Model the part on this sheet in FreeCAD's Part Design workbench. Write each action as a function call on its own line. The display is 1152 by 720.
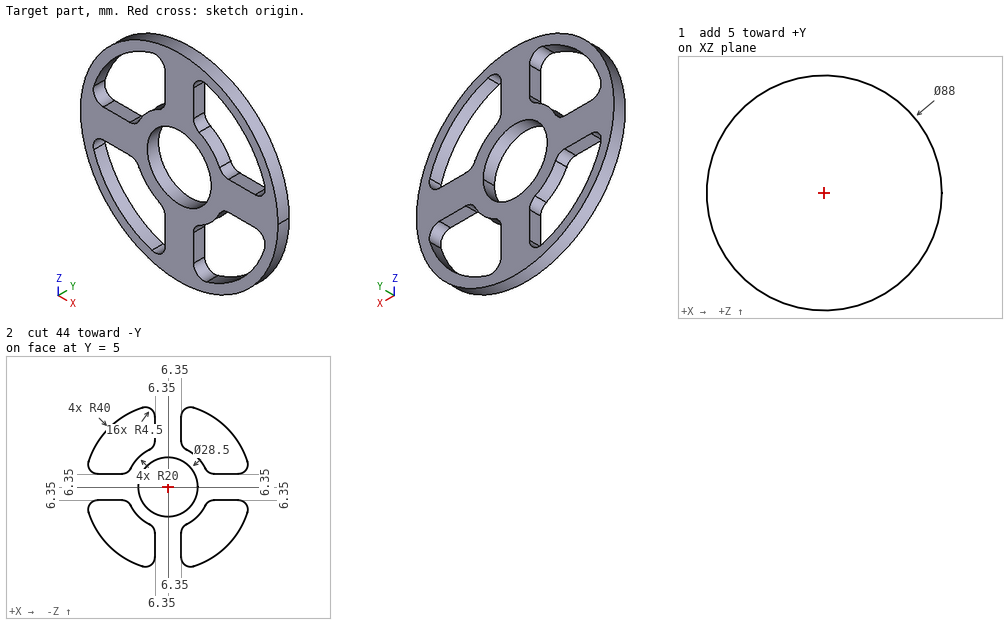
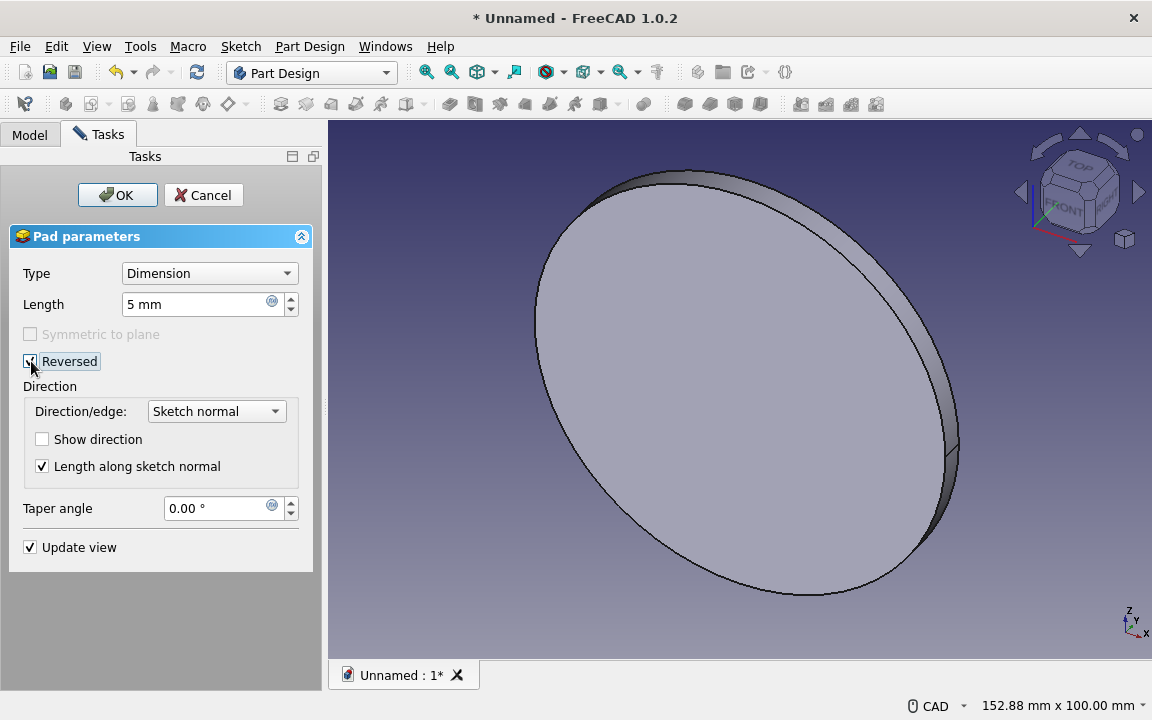
click(118, 195)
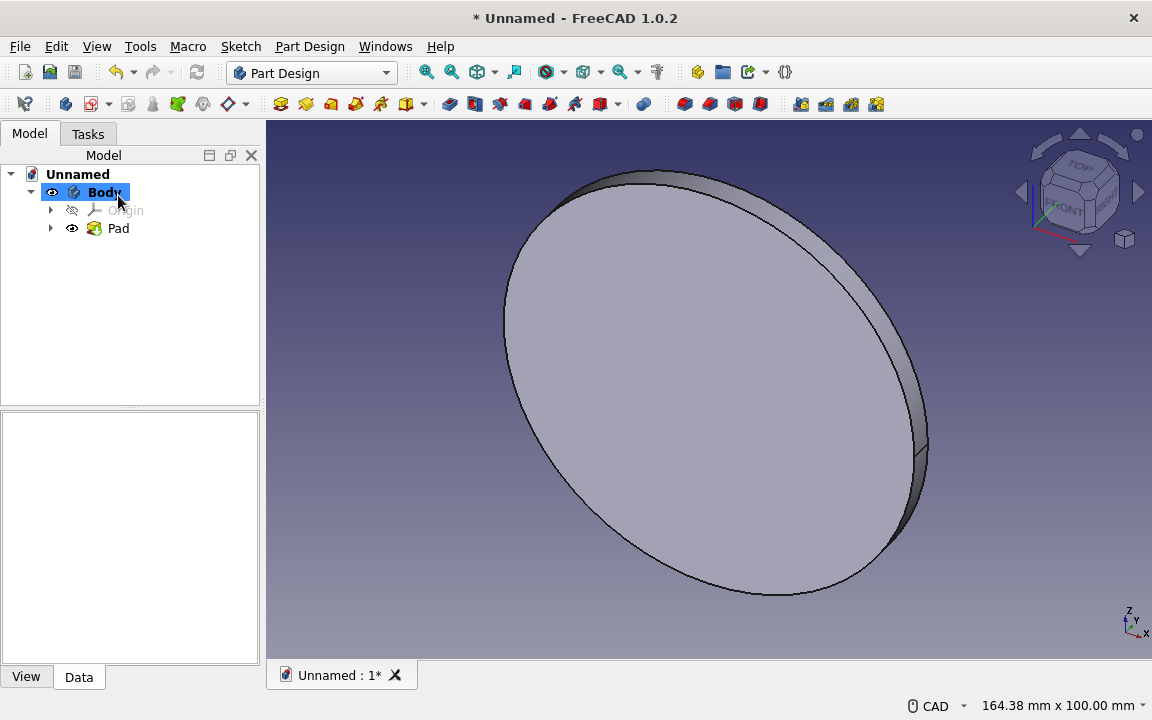
key(v)
key(f)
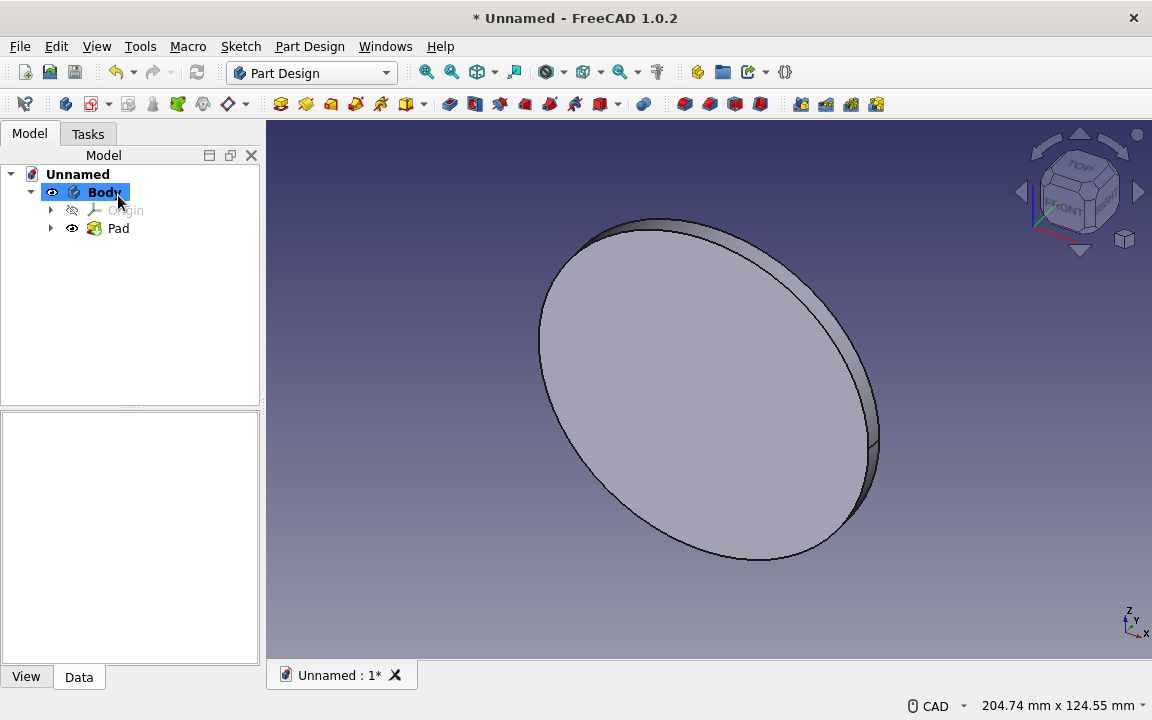
key(4)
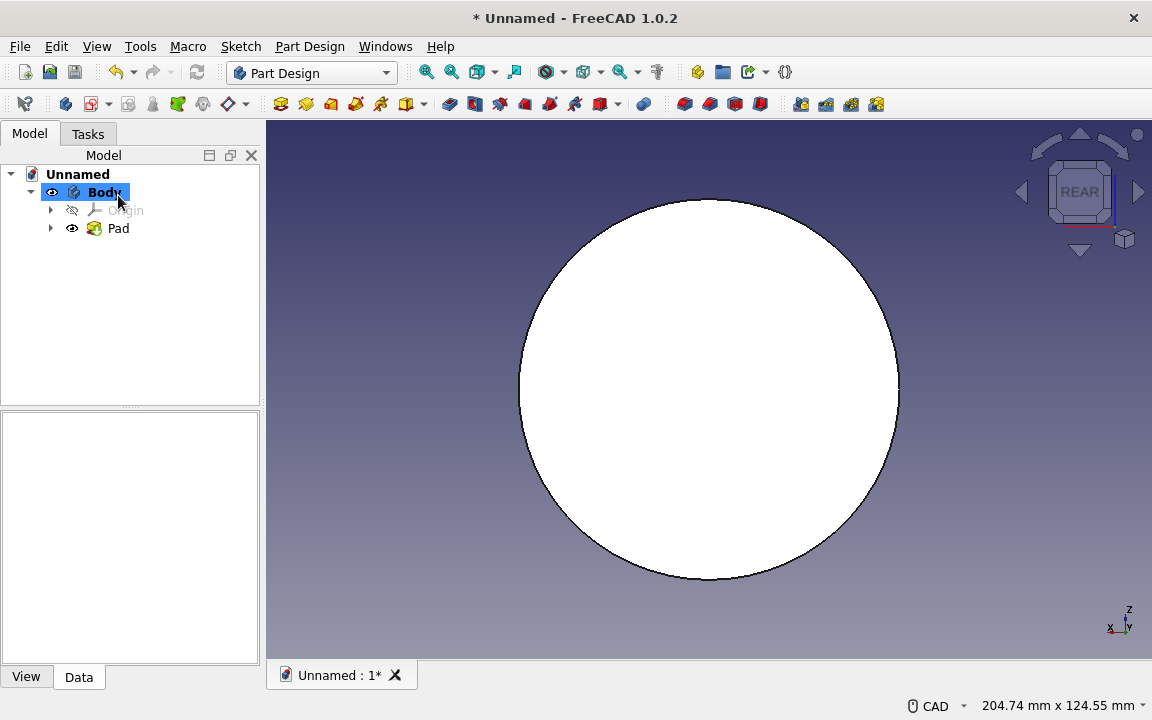
click(709, 388)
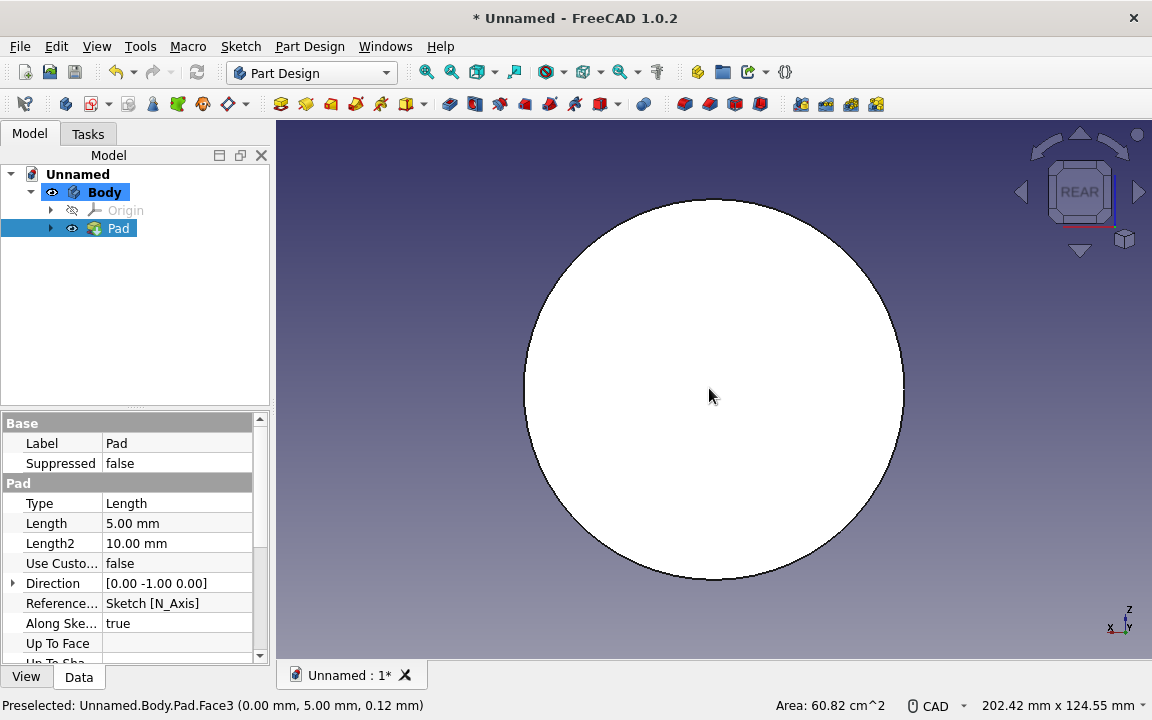
click(90, 104)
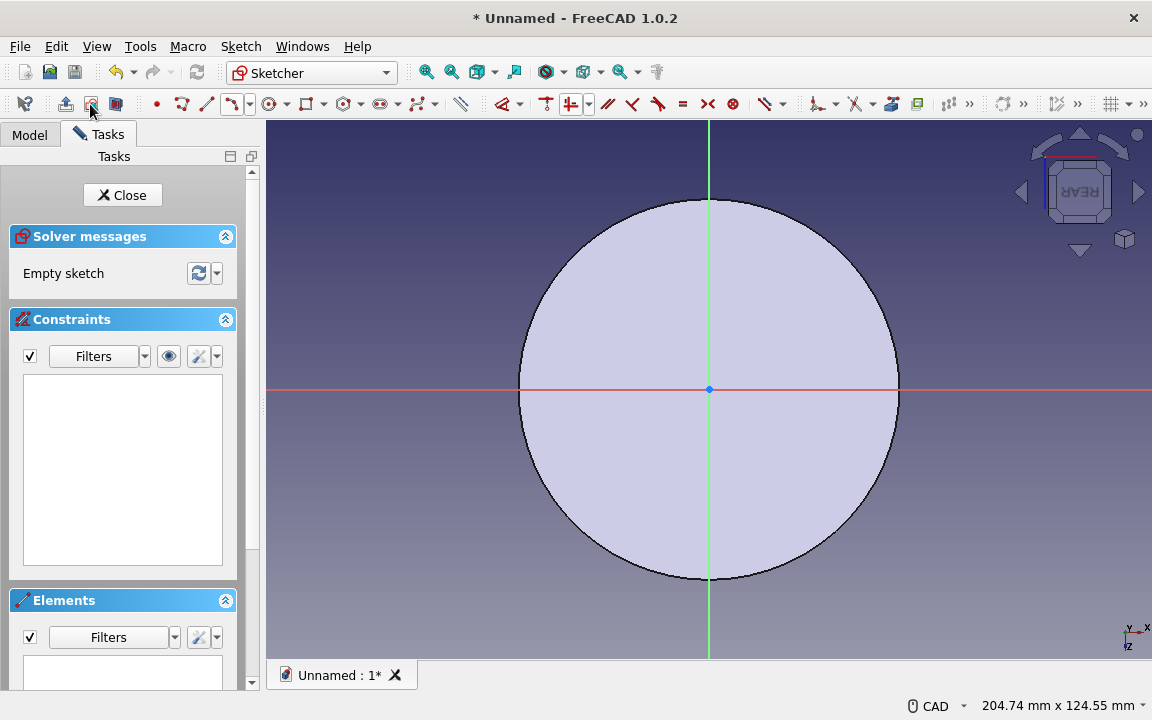
click(207, 104)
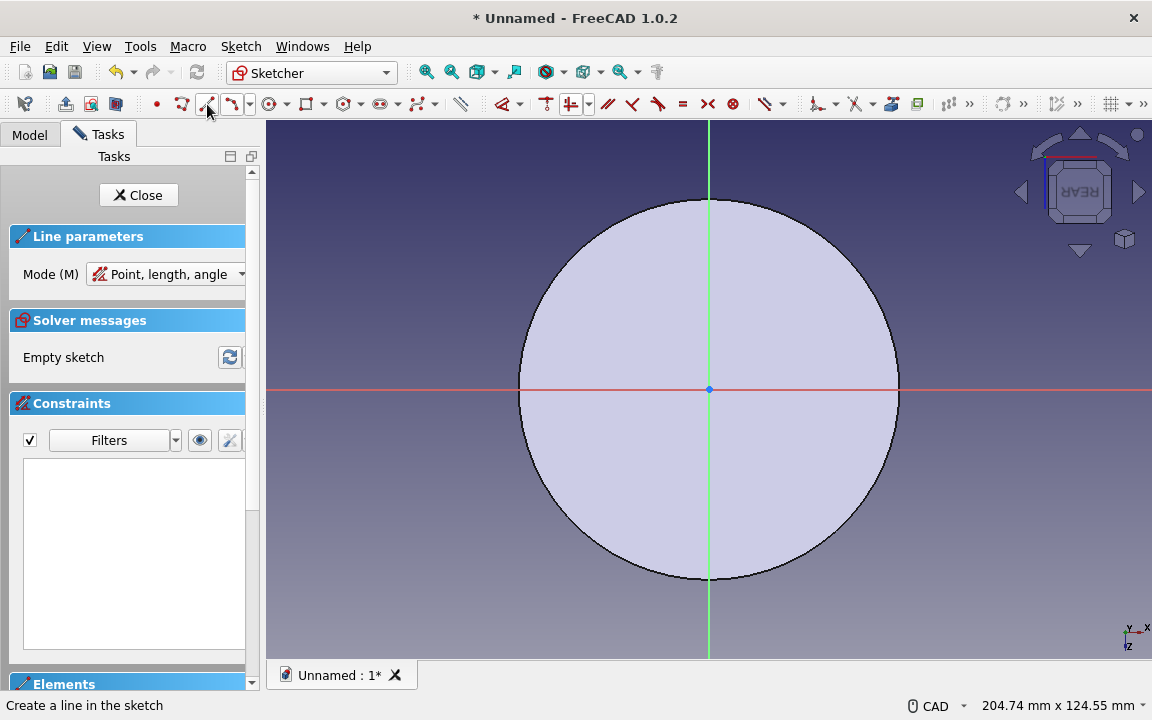
click(563, 362)
click(614, 362)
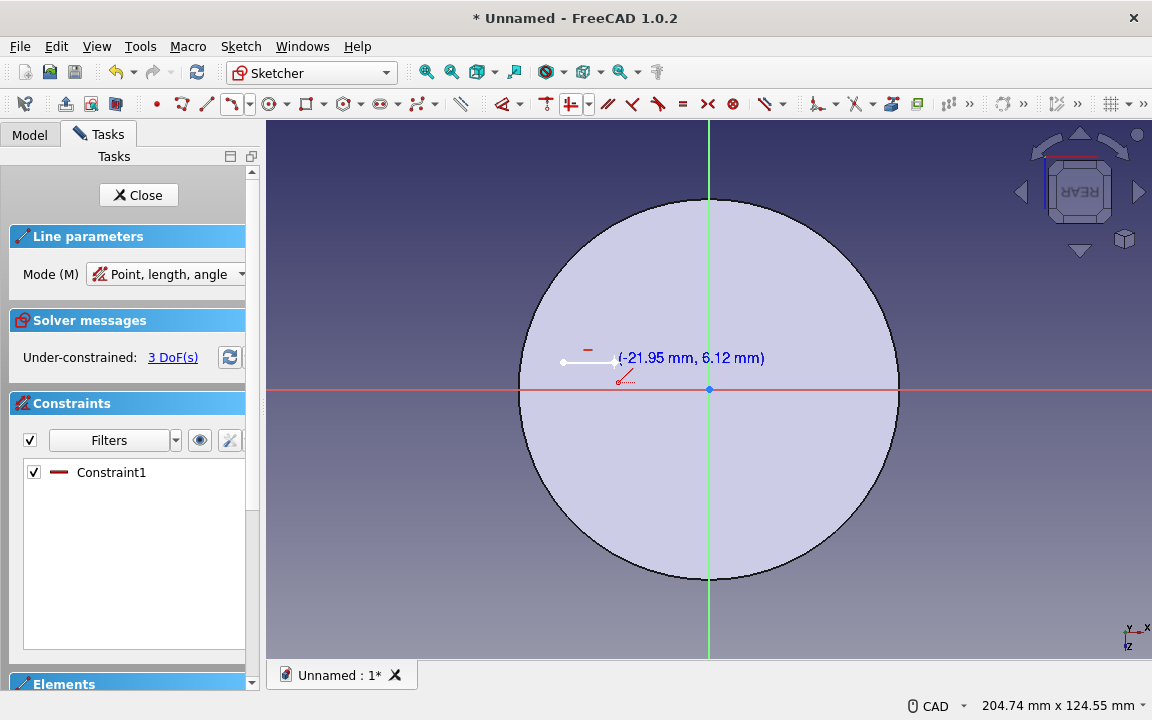
click(682, 294)
click(682, 243)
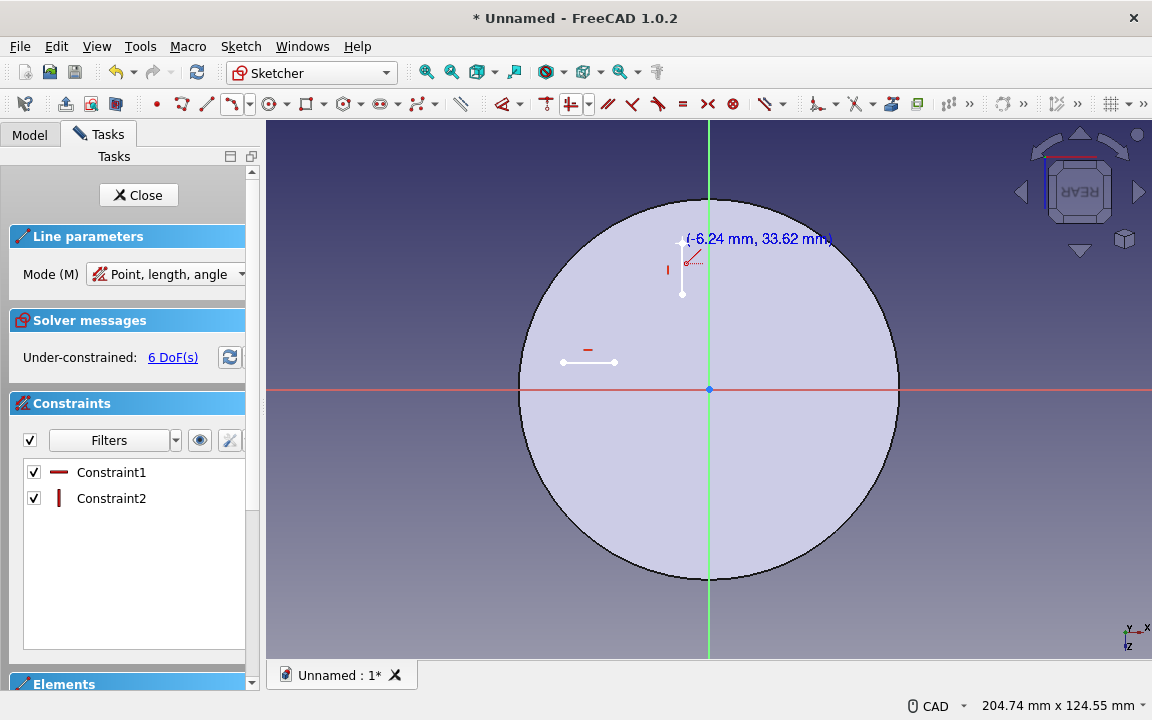
key(g)
key(3)
key(a)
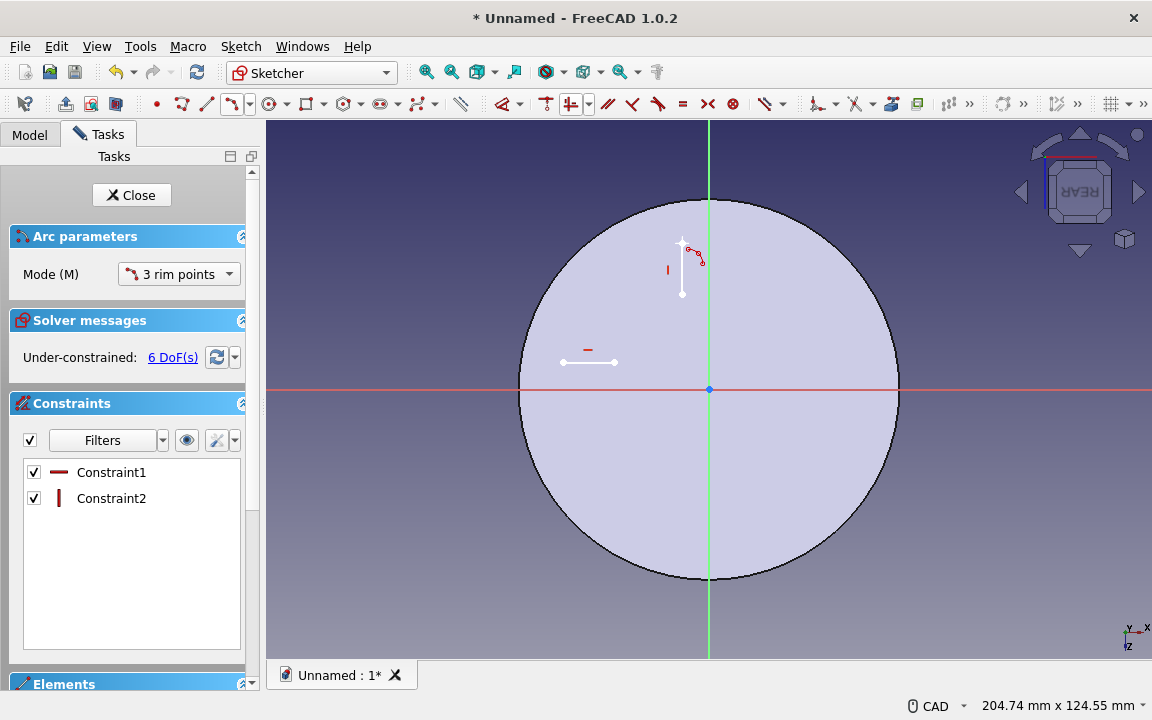
click(614, 363)
click(631, 351)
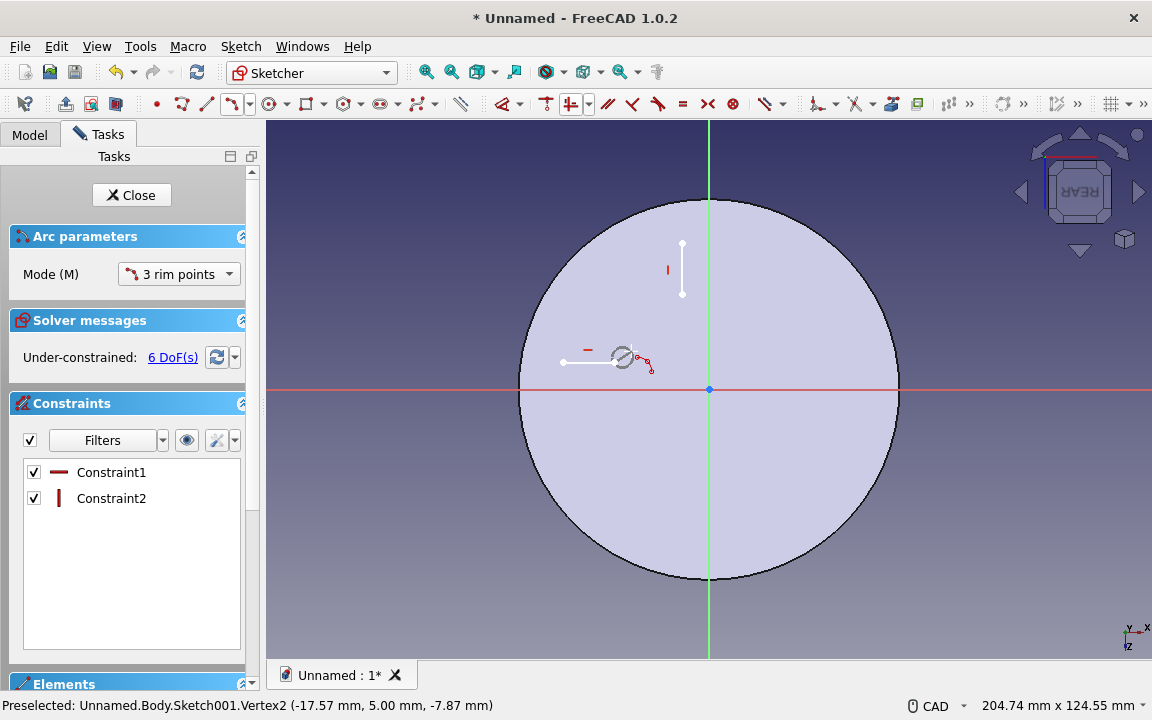
scroll(624, 359, up, 9)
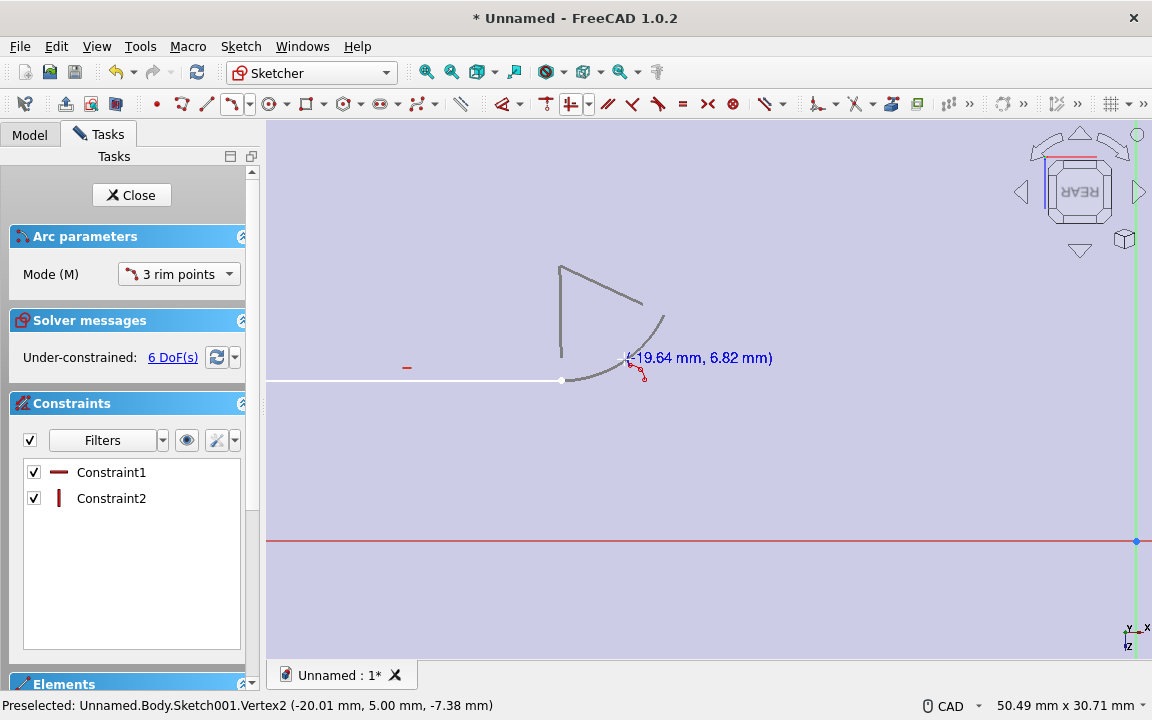
click(623, 357)